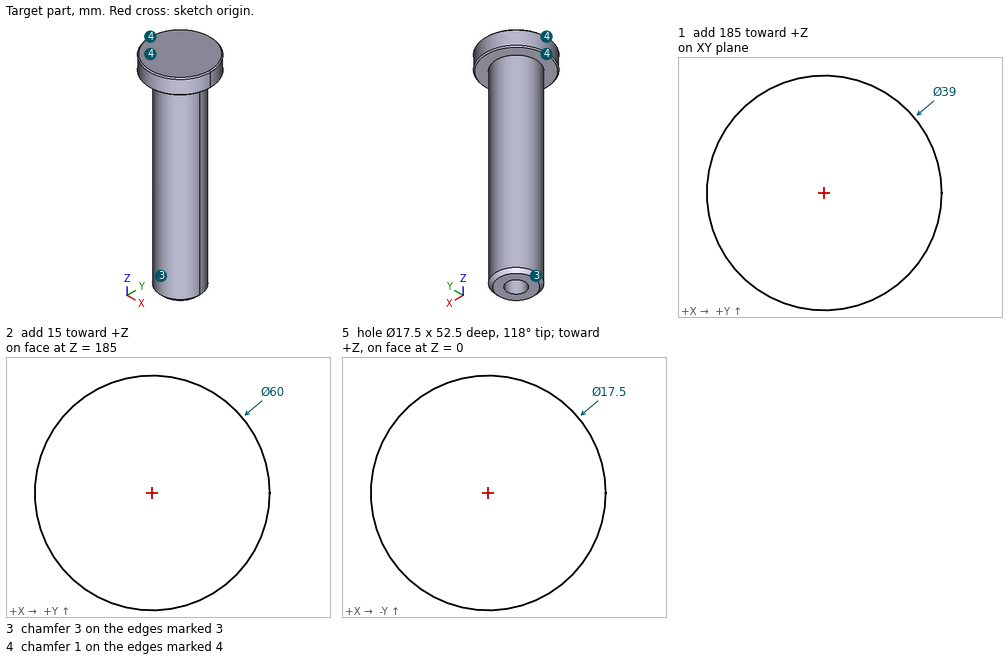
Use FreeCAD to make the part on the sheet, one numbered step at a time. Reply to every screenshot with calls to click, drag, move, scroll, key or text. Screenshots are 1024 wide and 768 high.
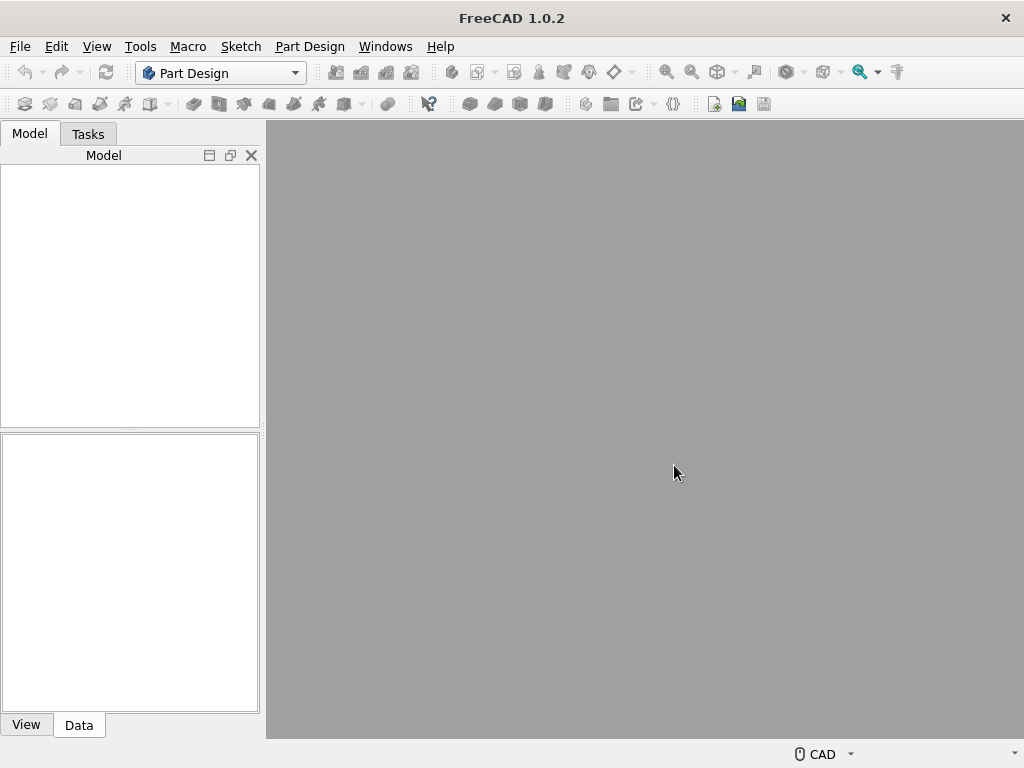
click(714, 104)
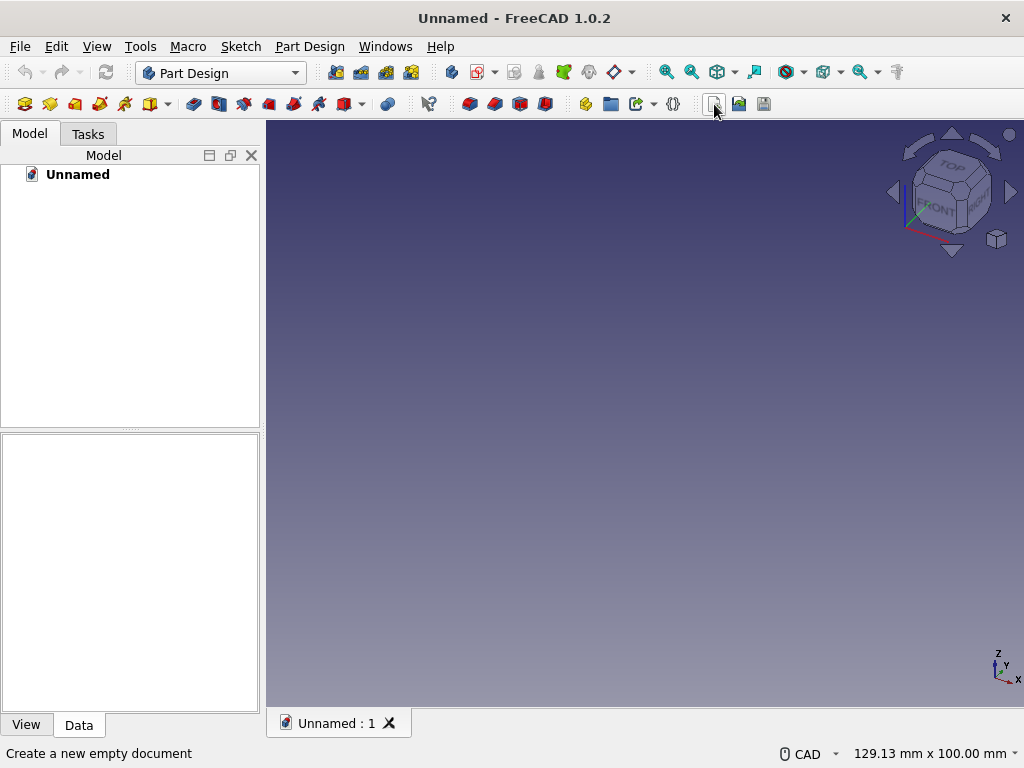
click(476, 72)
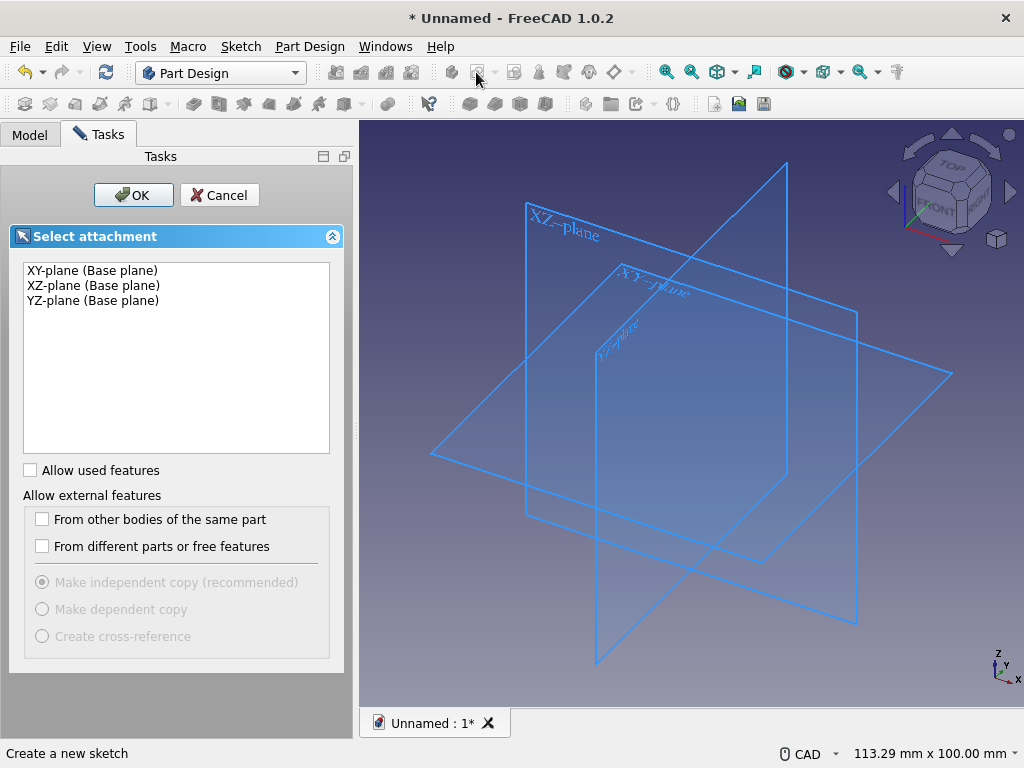
click(84, 270)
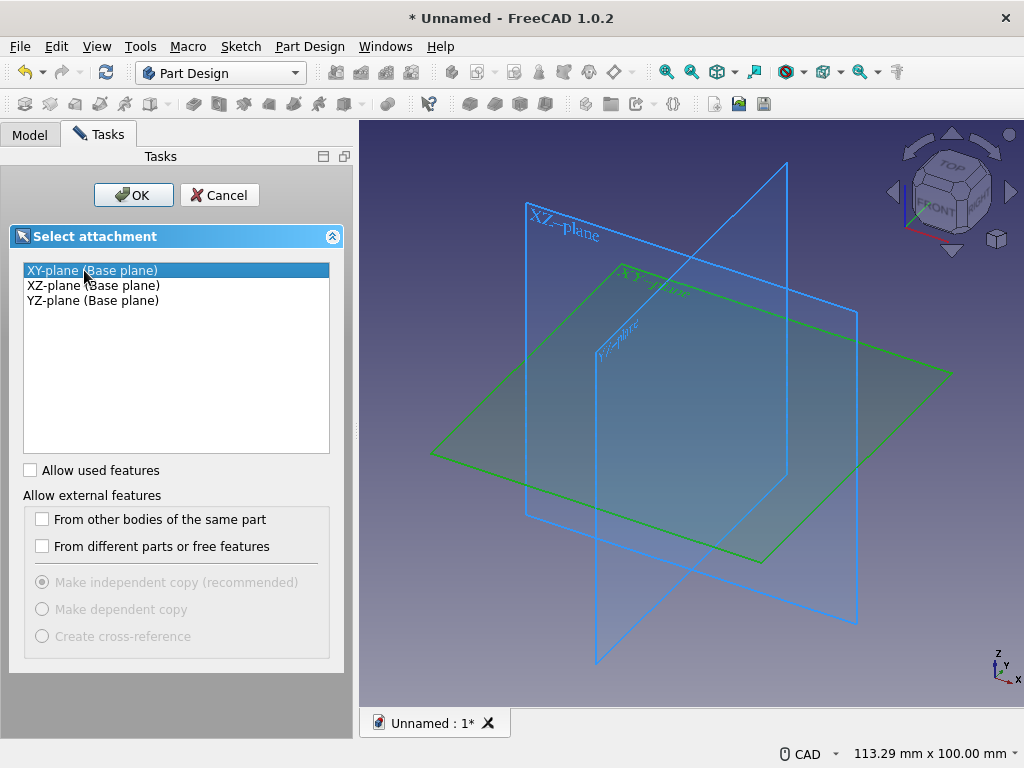
click(134, 195)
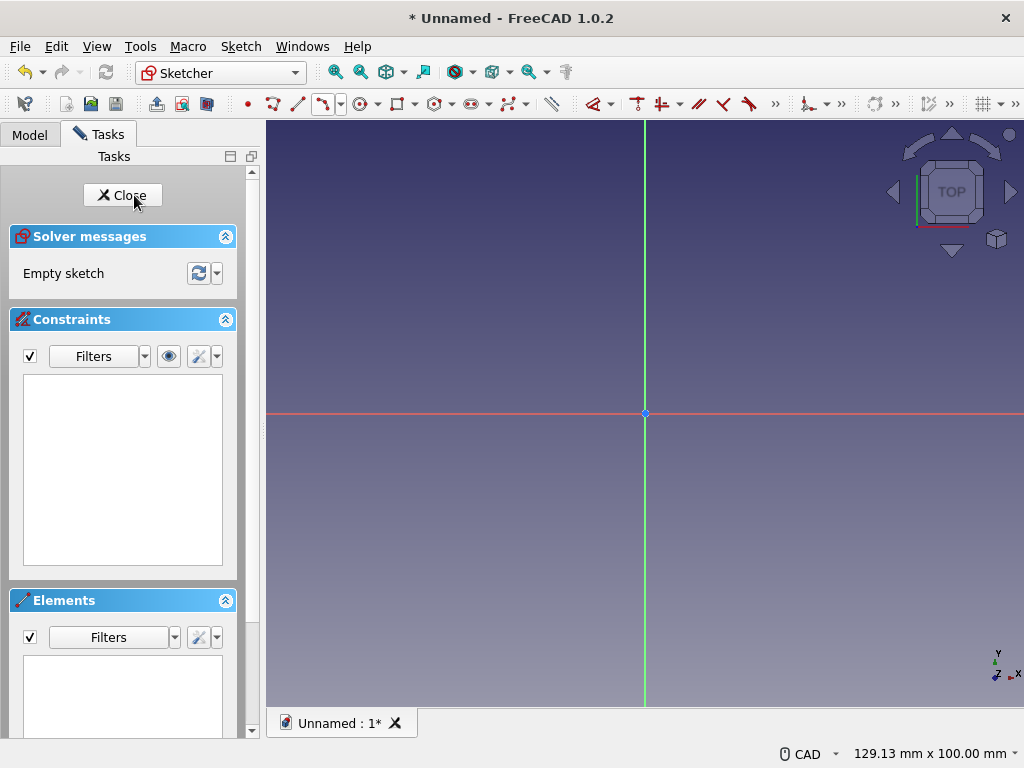
scroll(784, 413, up, 2)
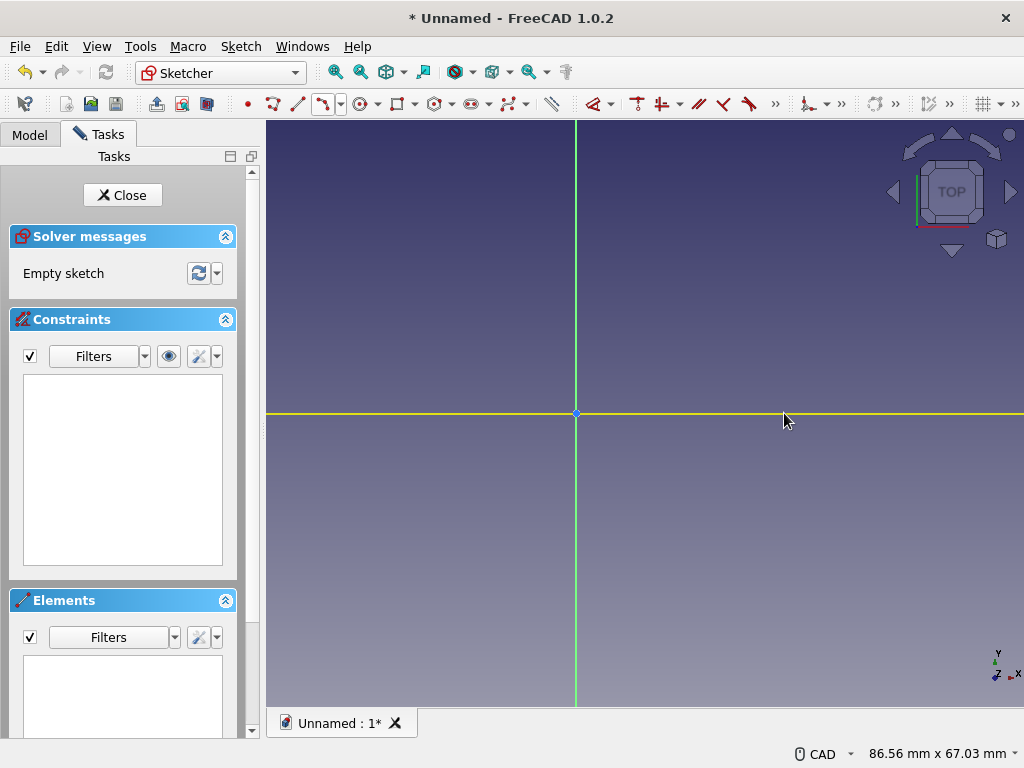
click(360, 104)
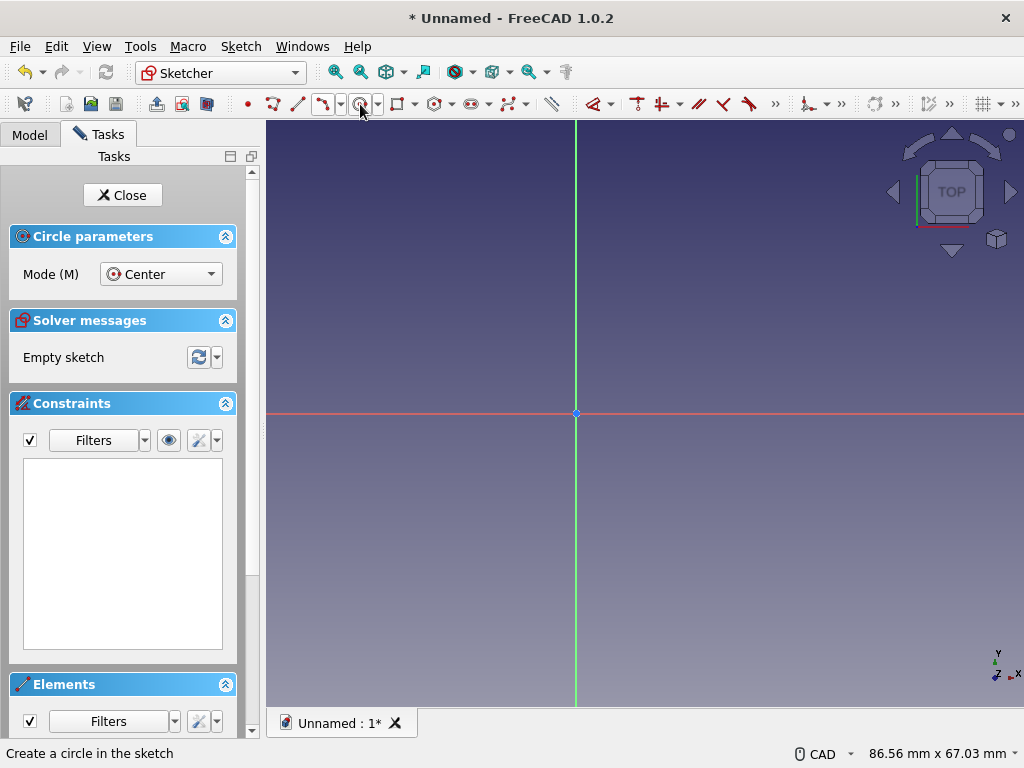
click(576, 414)
click(697, 293)
key(Escape)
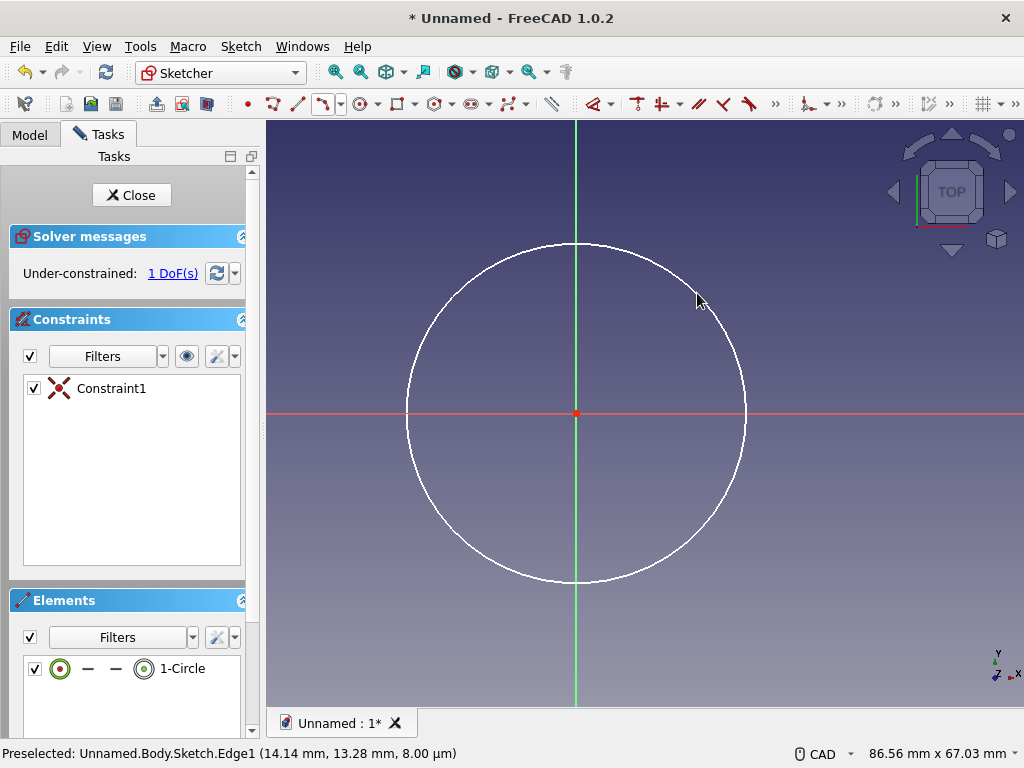
click(592, 104)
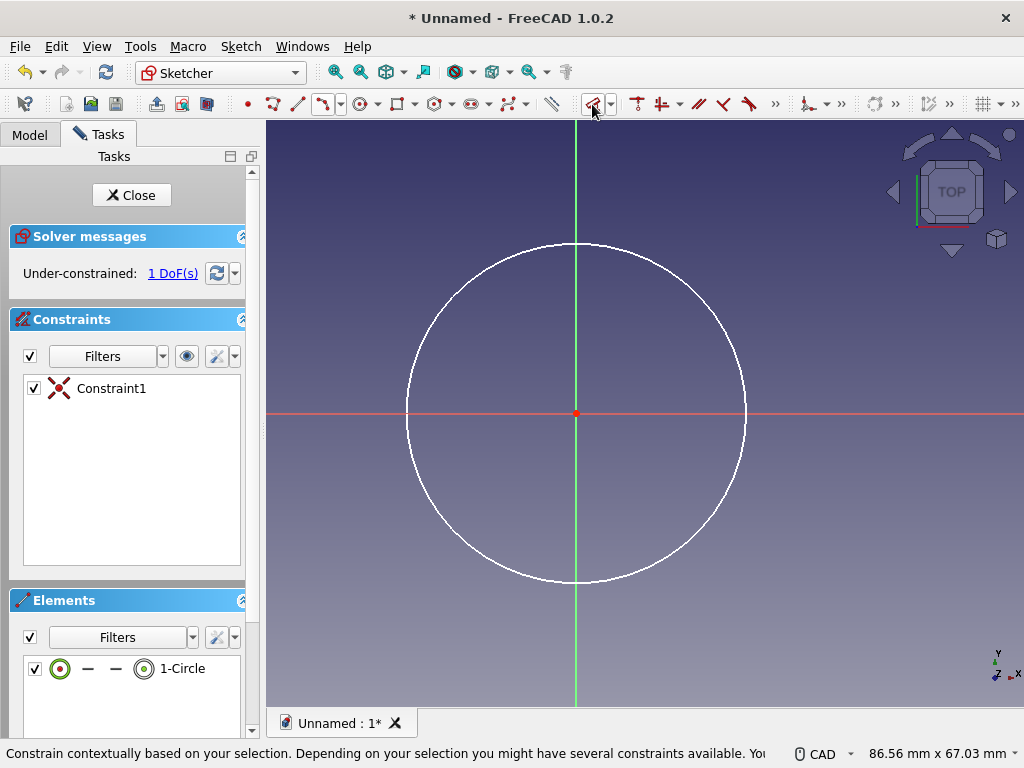
click(696, 293)
click(719, 270)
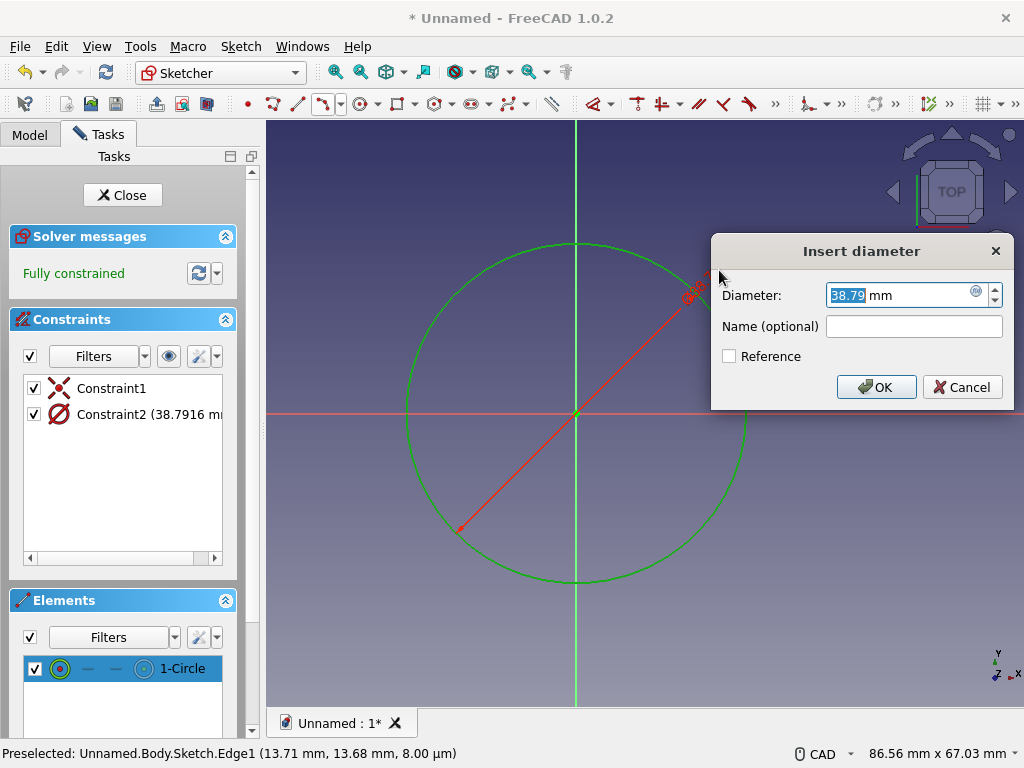
text(39)
key(Return)
key(Escape)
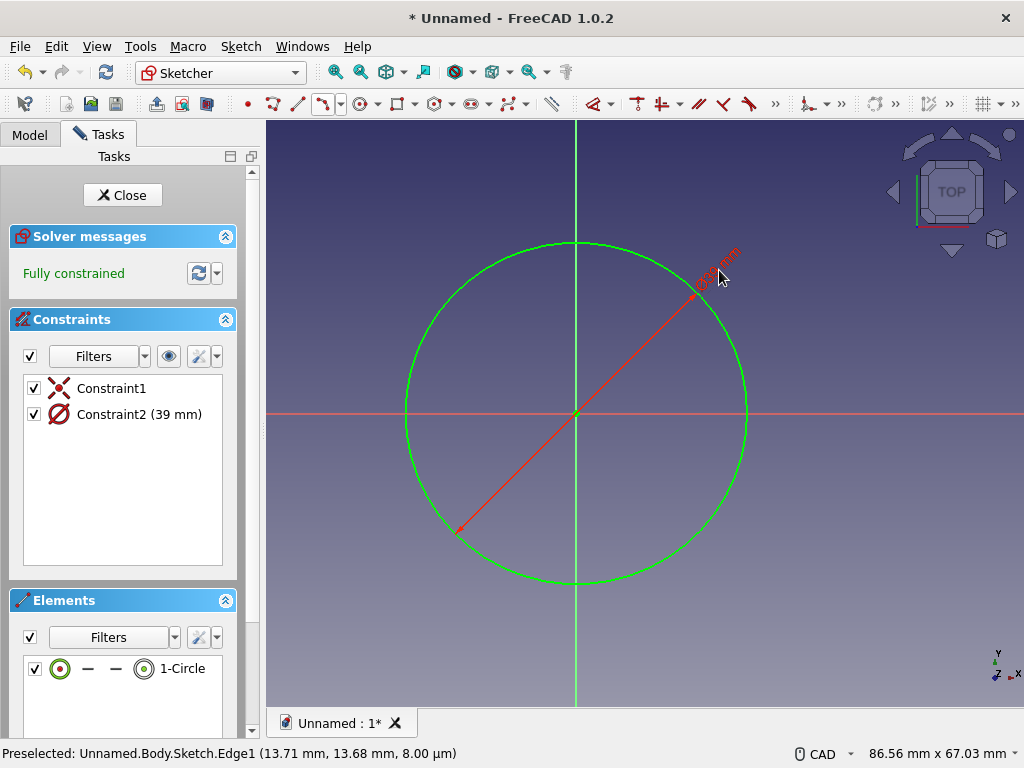
click(123, 195)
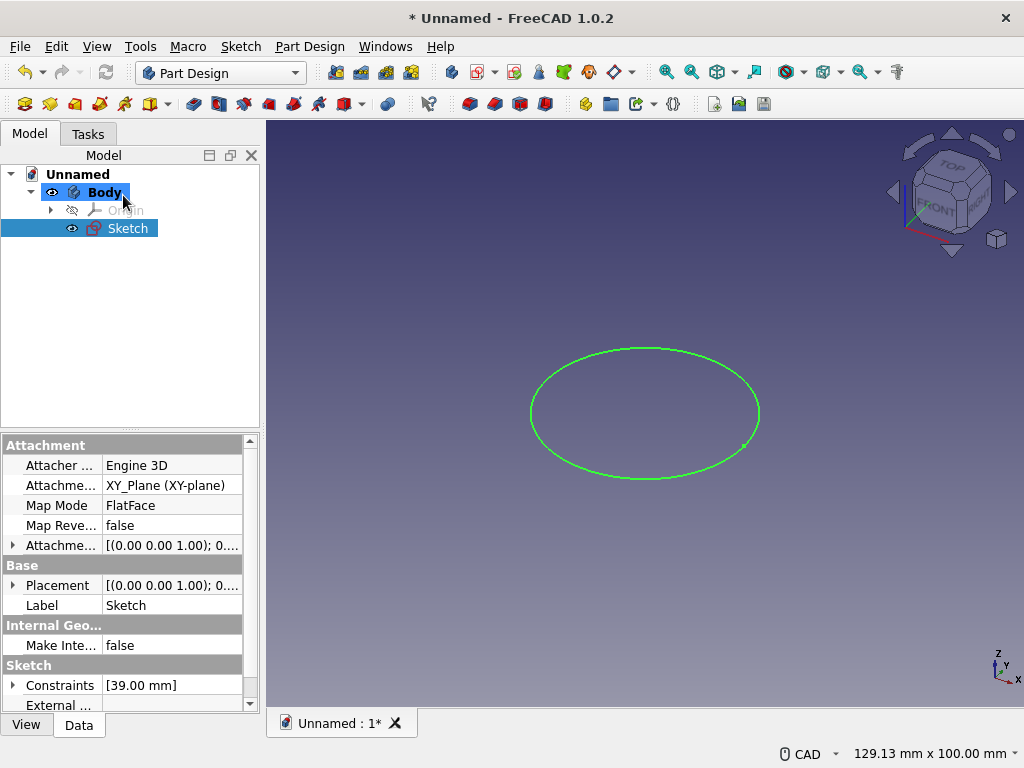
click(25, 104)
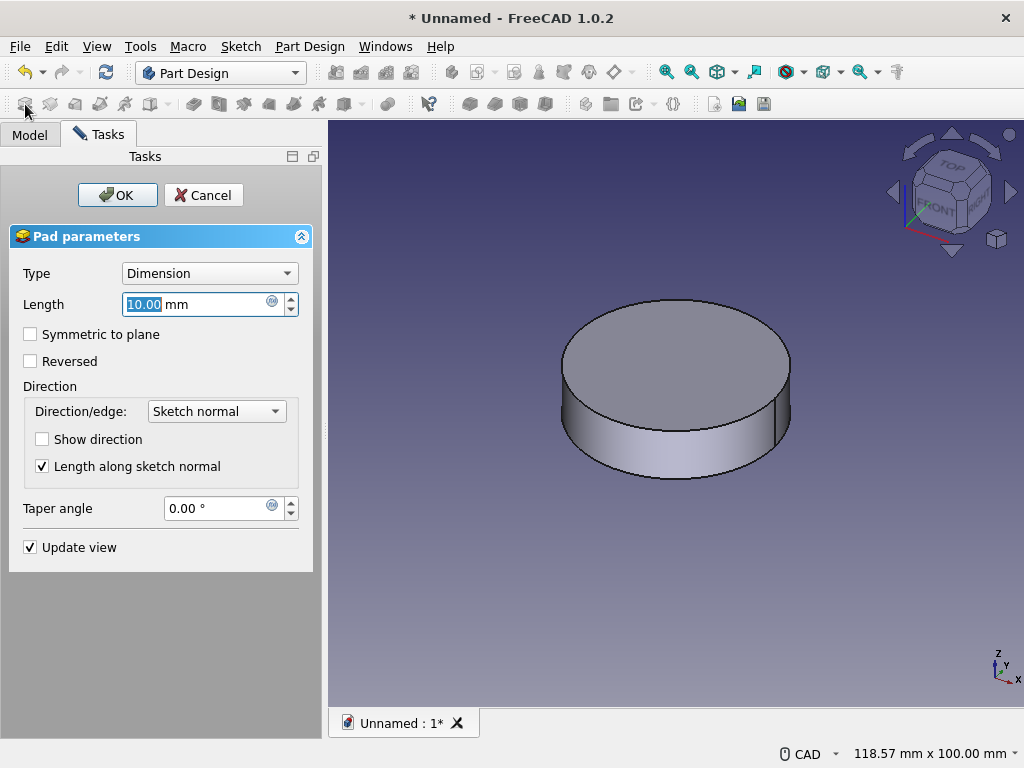
text(185)
key(Tab)